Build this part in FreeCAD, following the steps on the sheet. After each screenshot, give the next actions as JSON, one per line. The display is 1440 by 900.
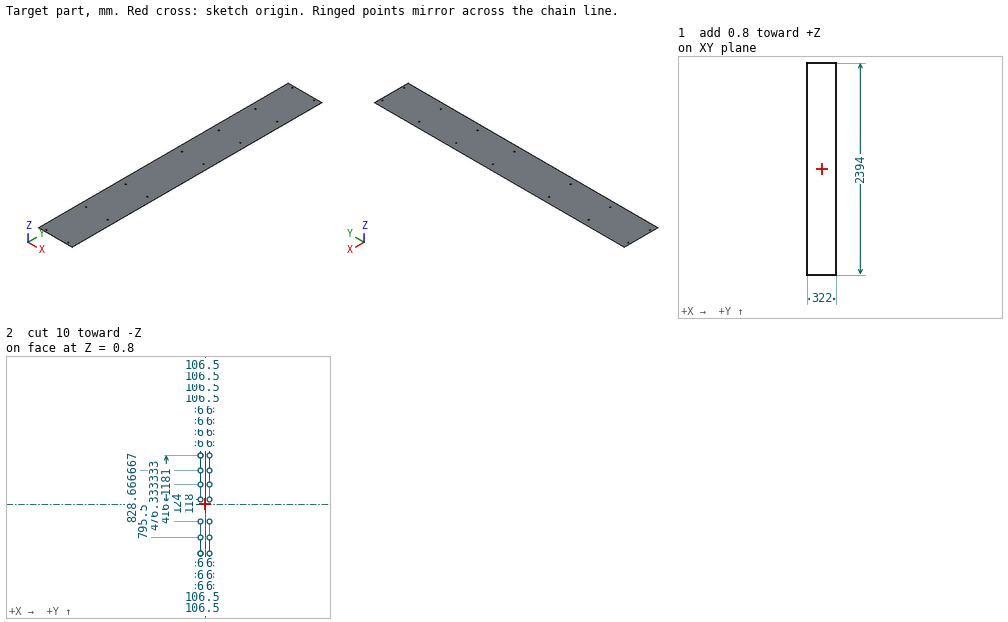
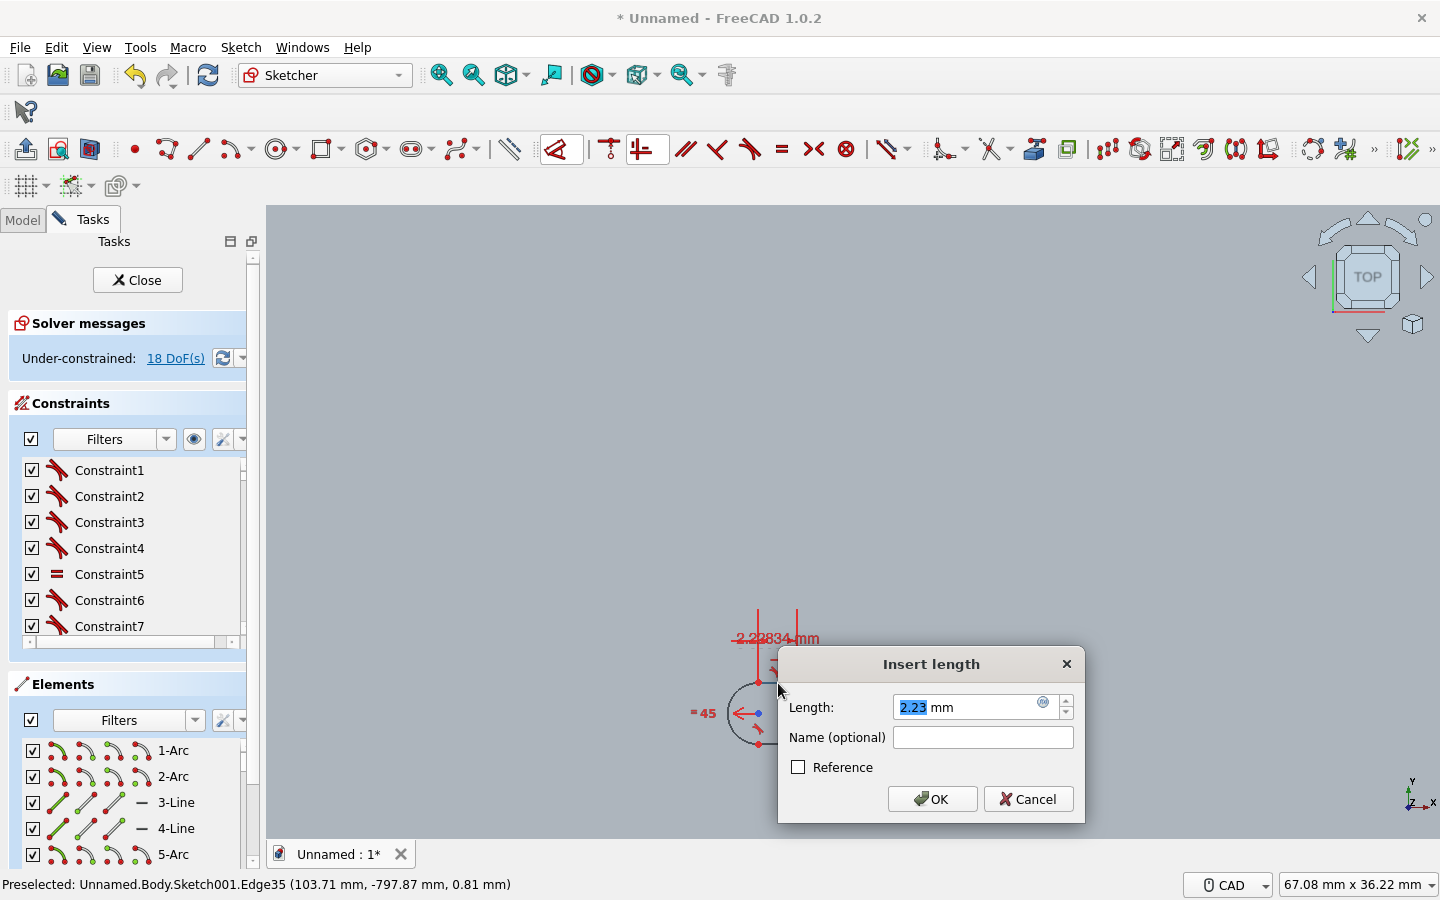
{"action": "type", "text": "6"}
{"action": "key", "text": "Return"}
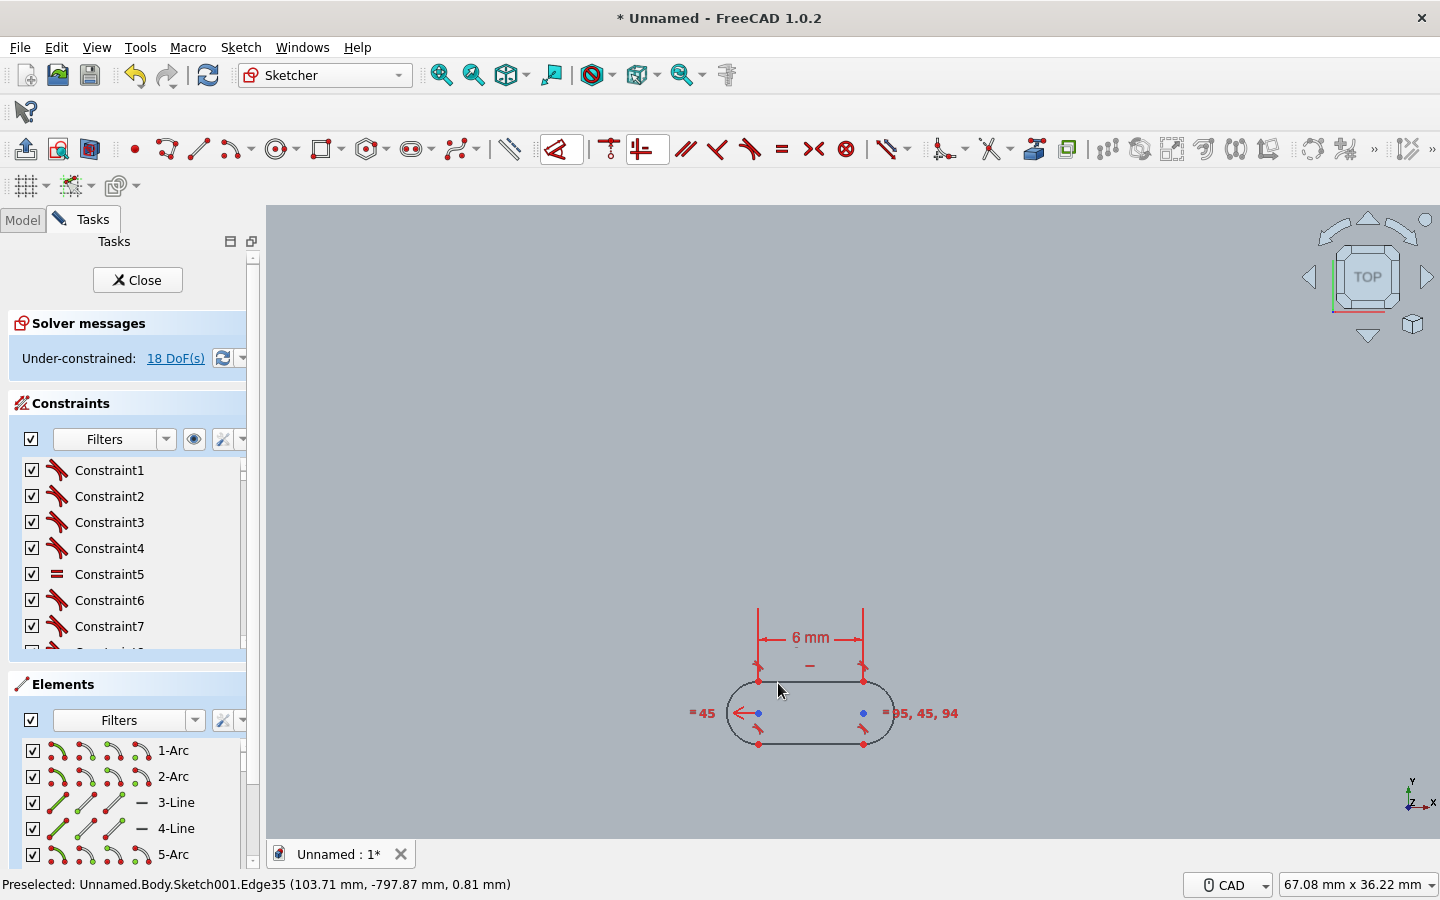
{"action": "scroll", "coordinate": [784, 522], "scroll_direction": "down", "scroll_amount": 15}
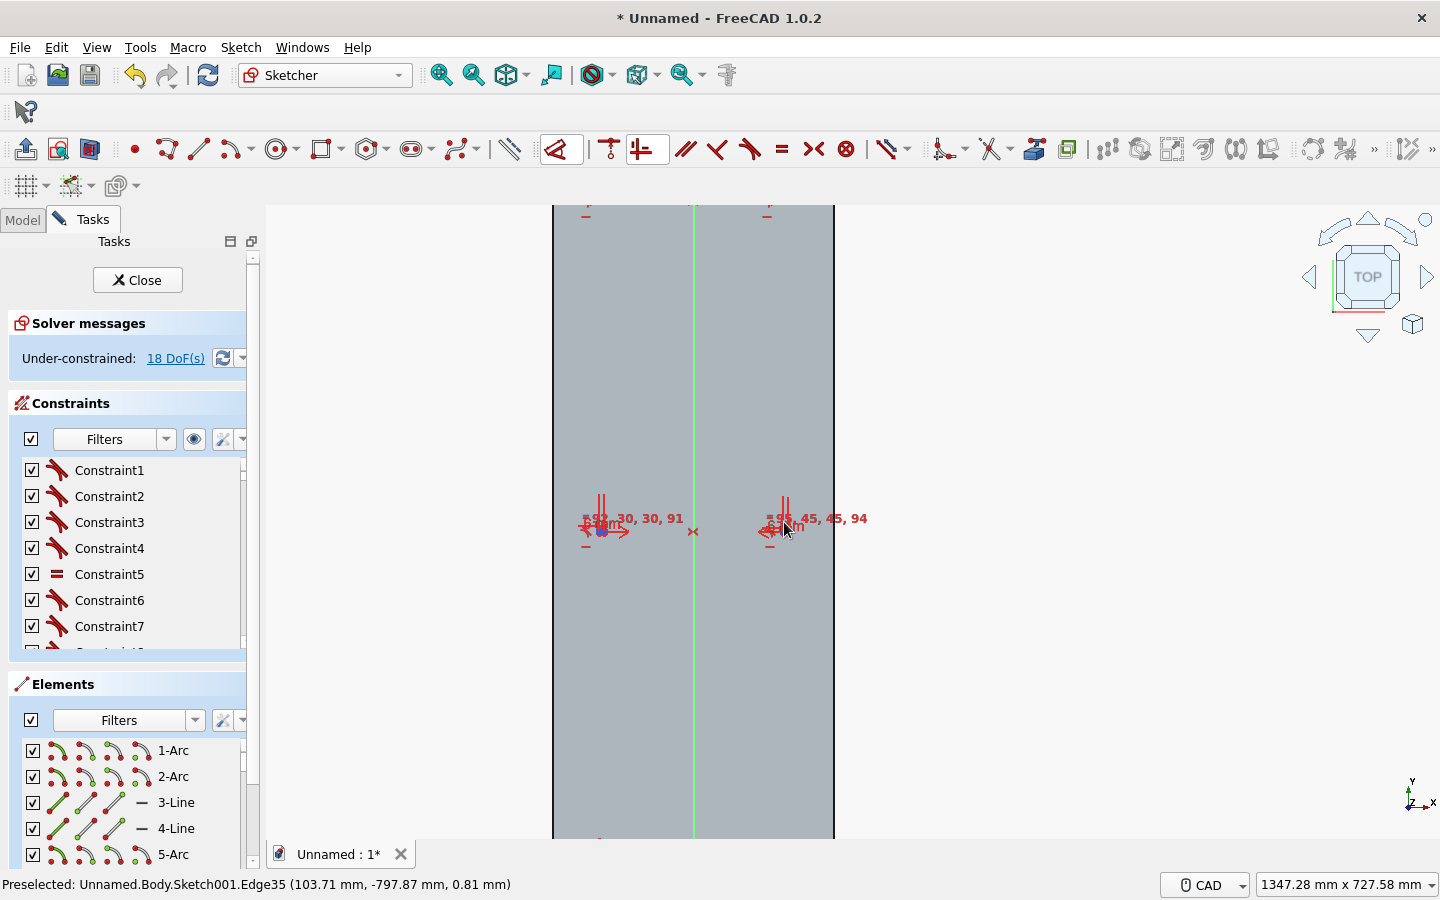
{"action": "scroll", "coordinate": [807, 696], "scroll_direction": "down", "scroll_amount": 8}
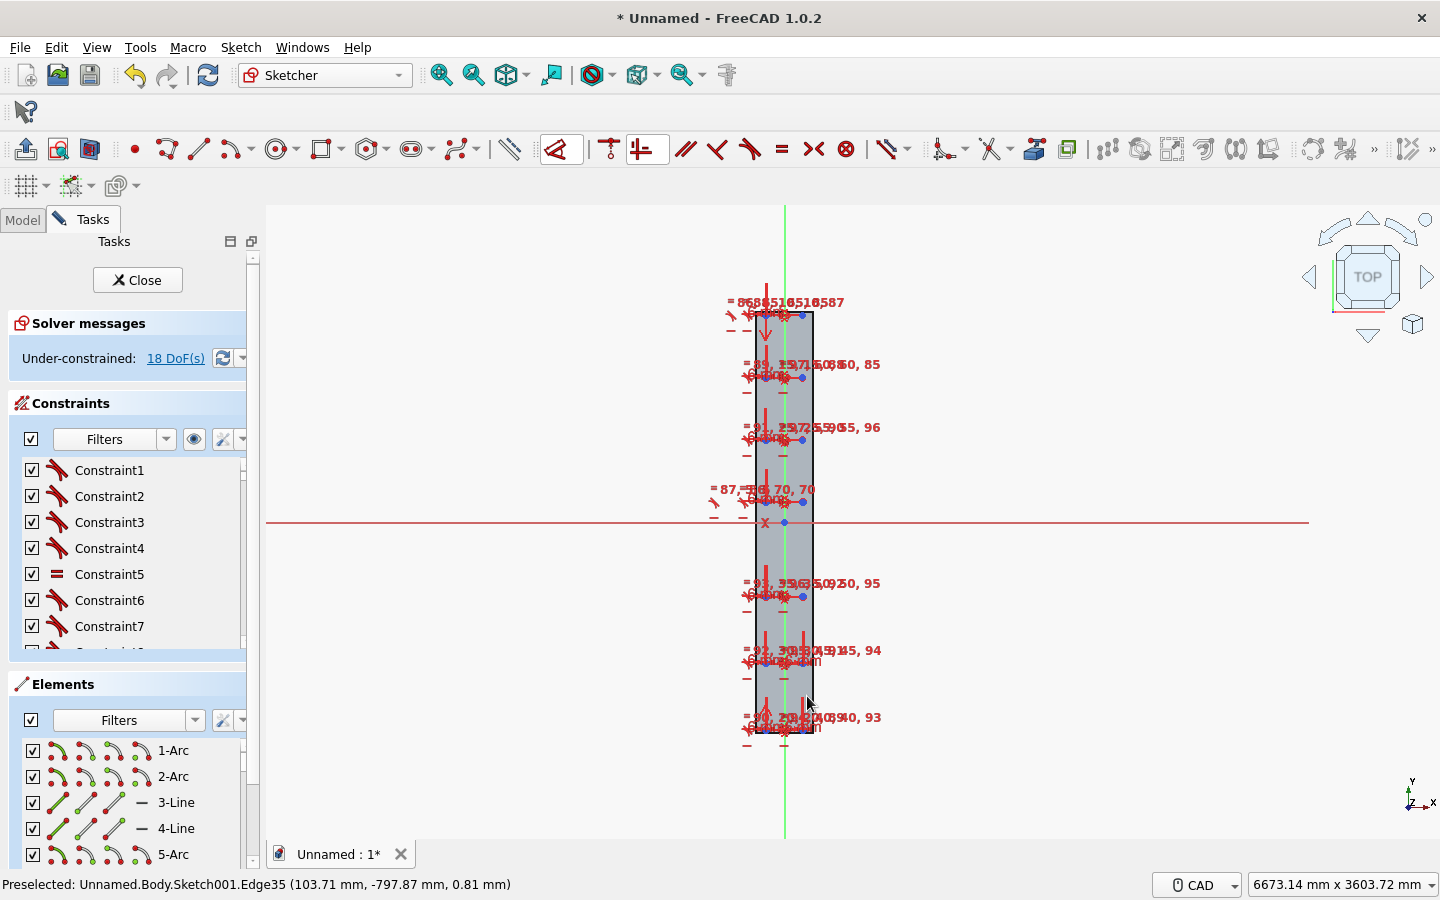
{"action": "scroll", "coordinate": [803, 596], "scroll_direction": "up", "scroll_amount": 19}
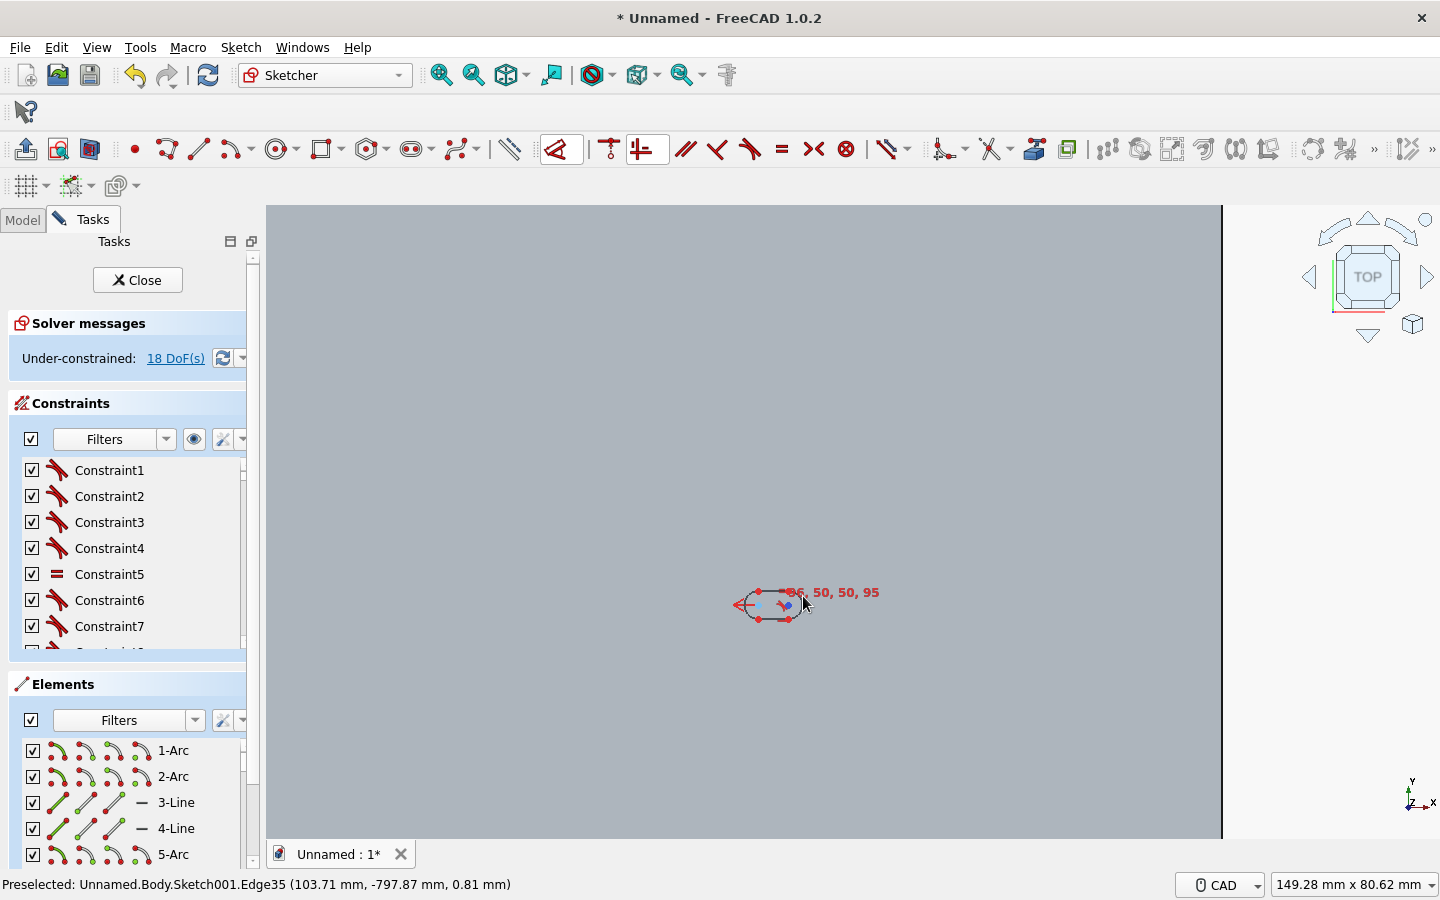
{"action": "left_click", "coordinate": [767, 591]}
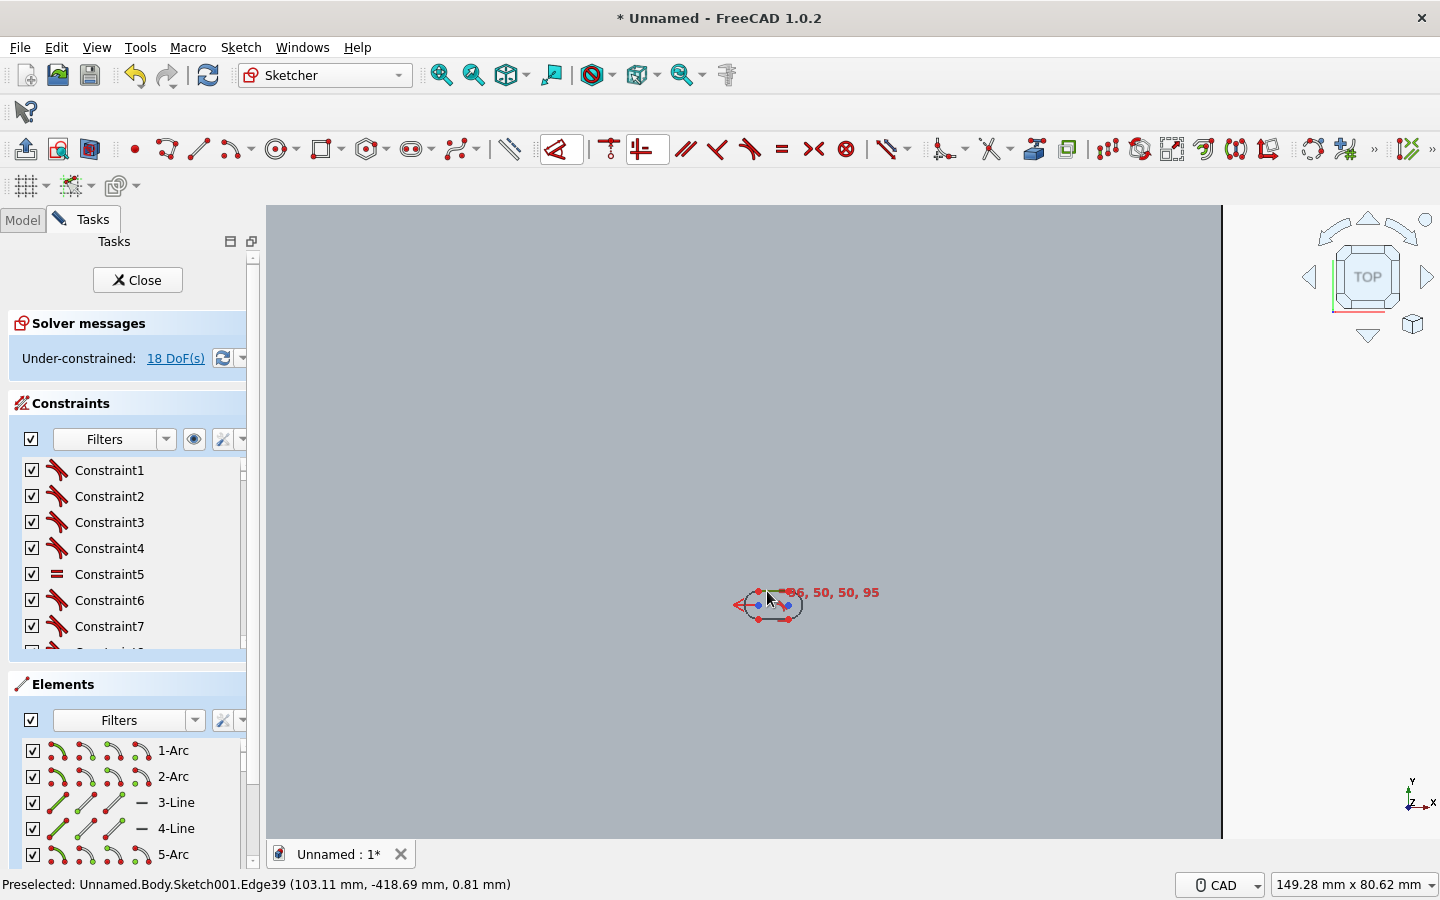
{"action": "key", "text": "l"}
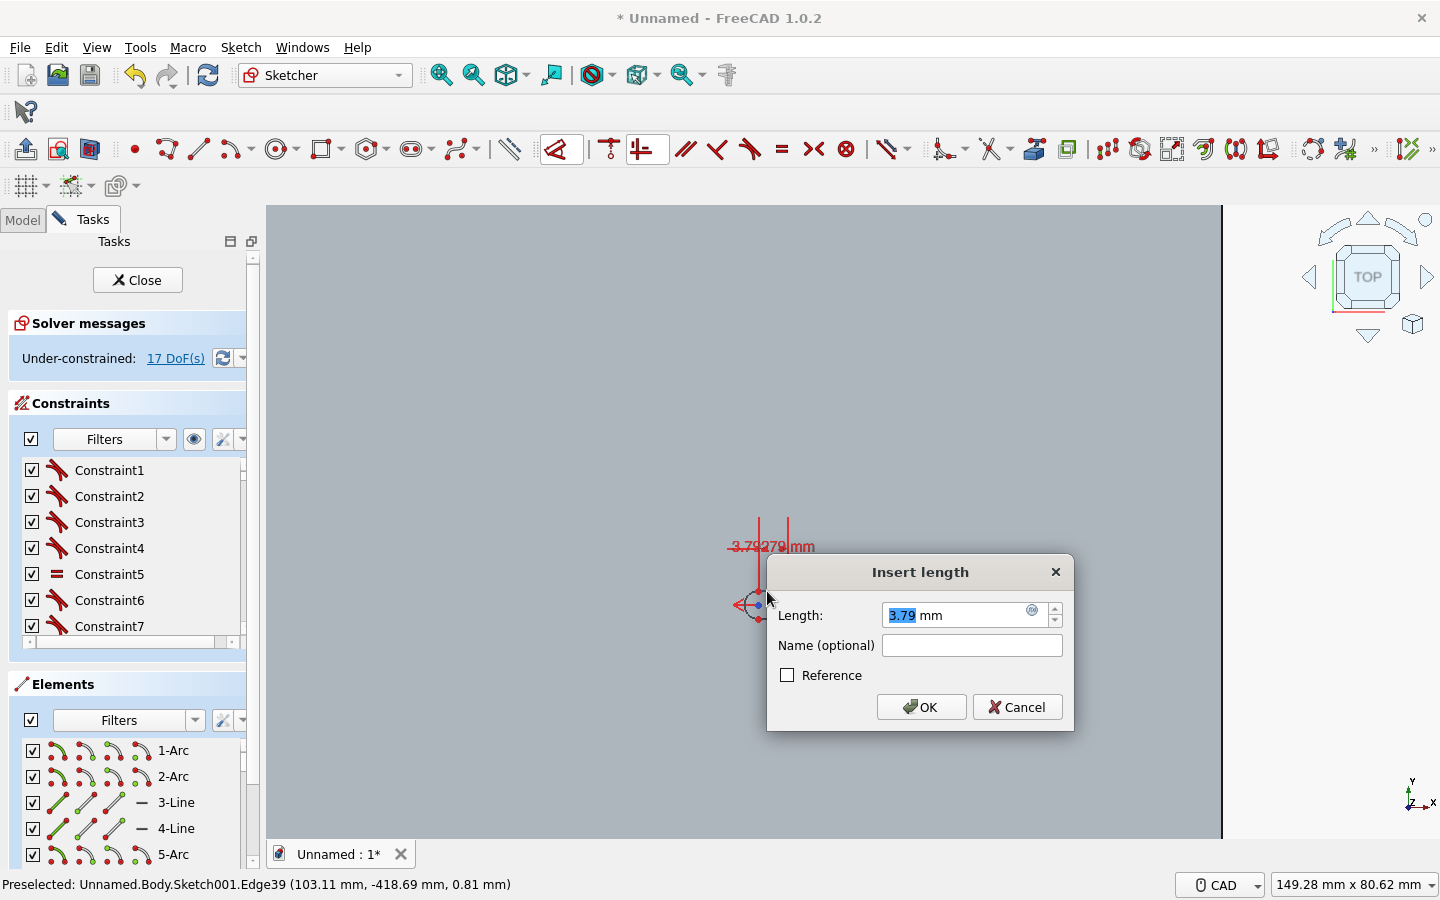
{"action": "type", "text": "6"}
{"action": "key", "text": "Return"}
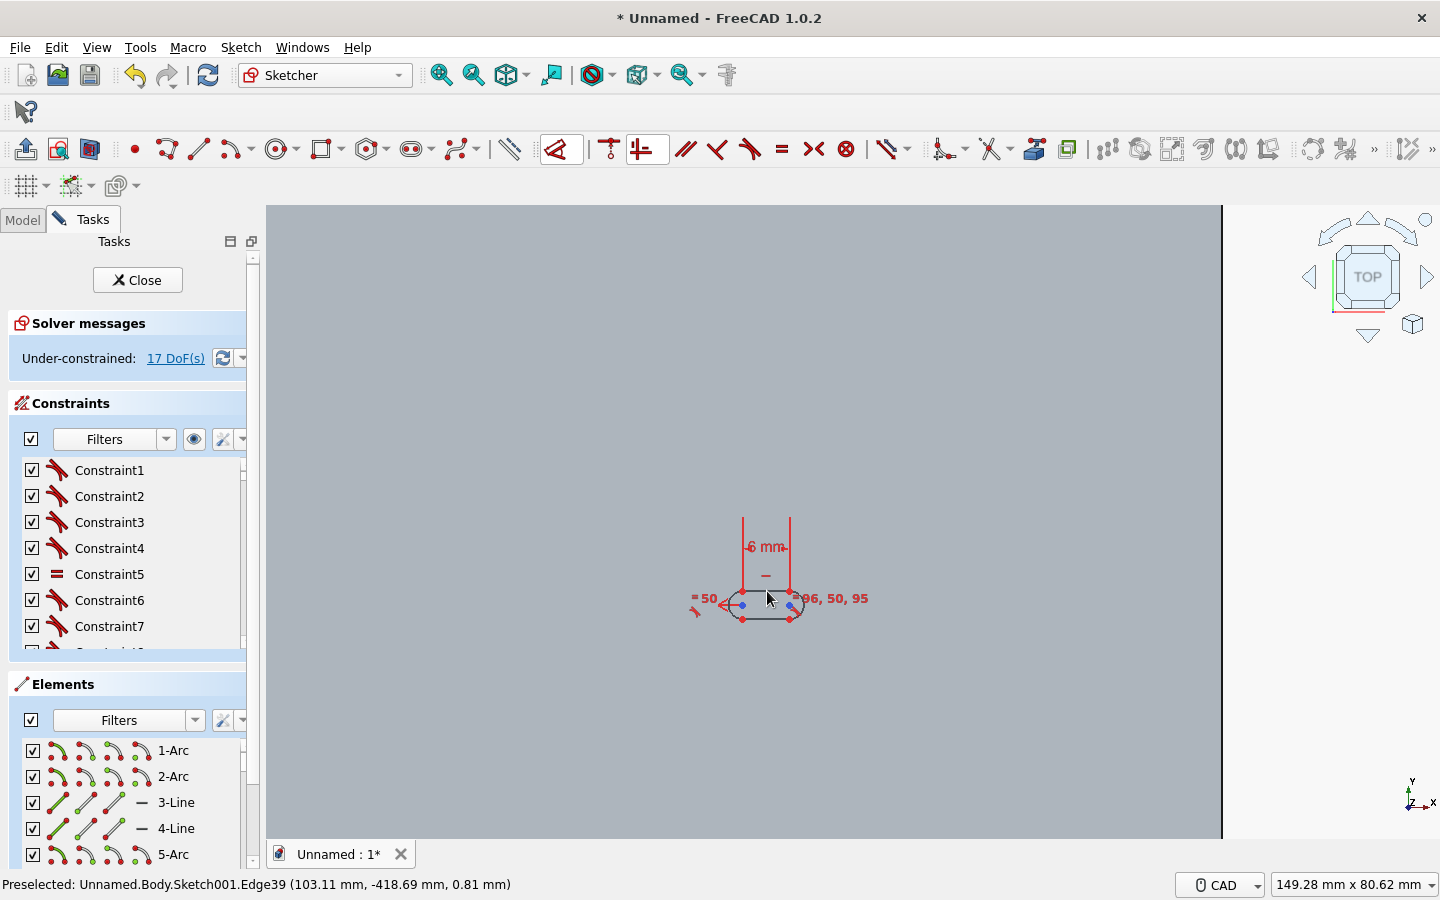
{"action": "scroll", "coordinate": [808, 613], "scroll_direction": "down", "scroll_amount": 18}